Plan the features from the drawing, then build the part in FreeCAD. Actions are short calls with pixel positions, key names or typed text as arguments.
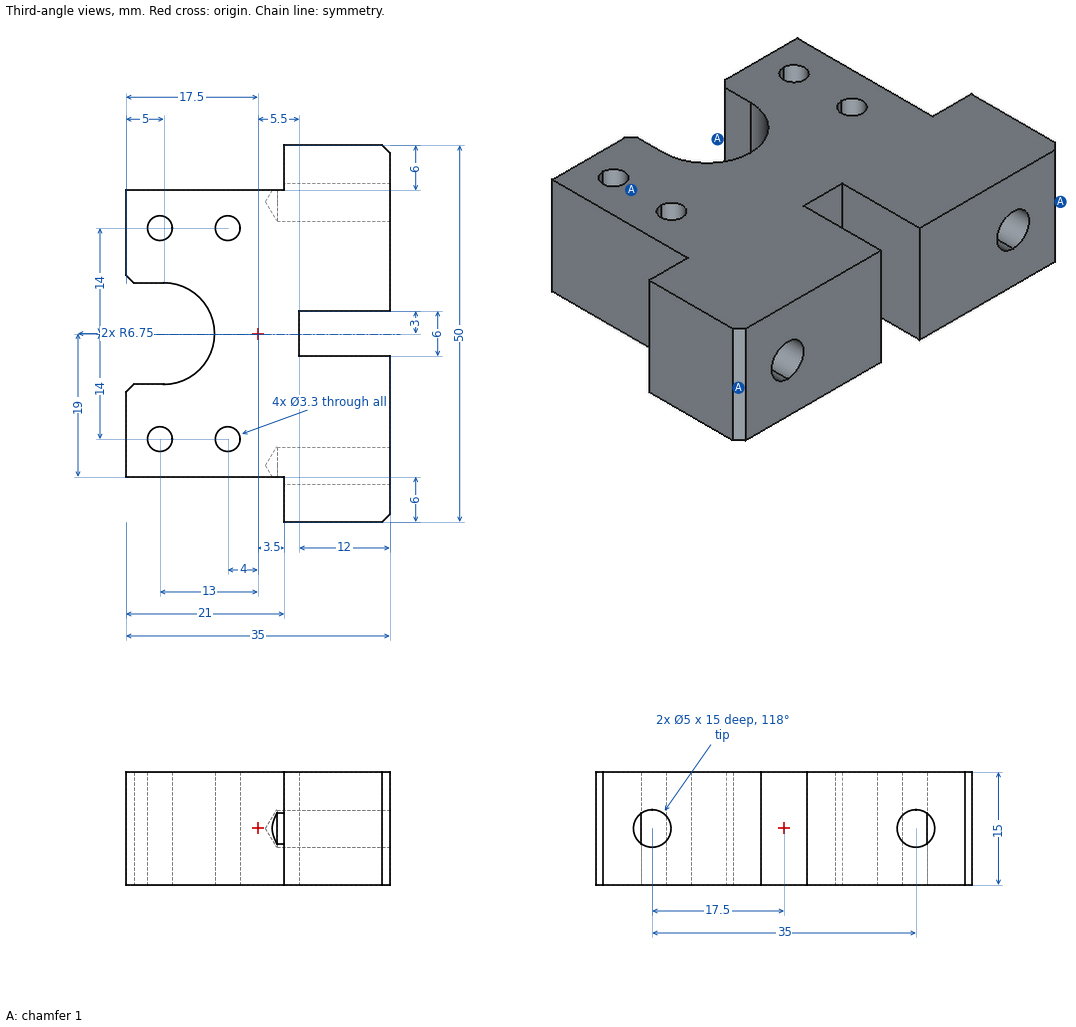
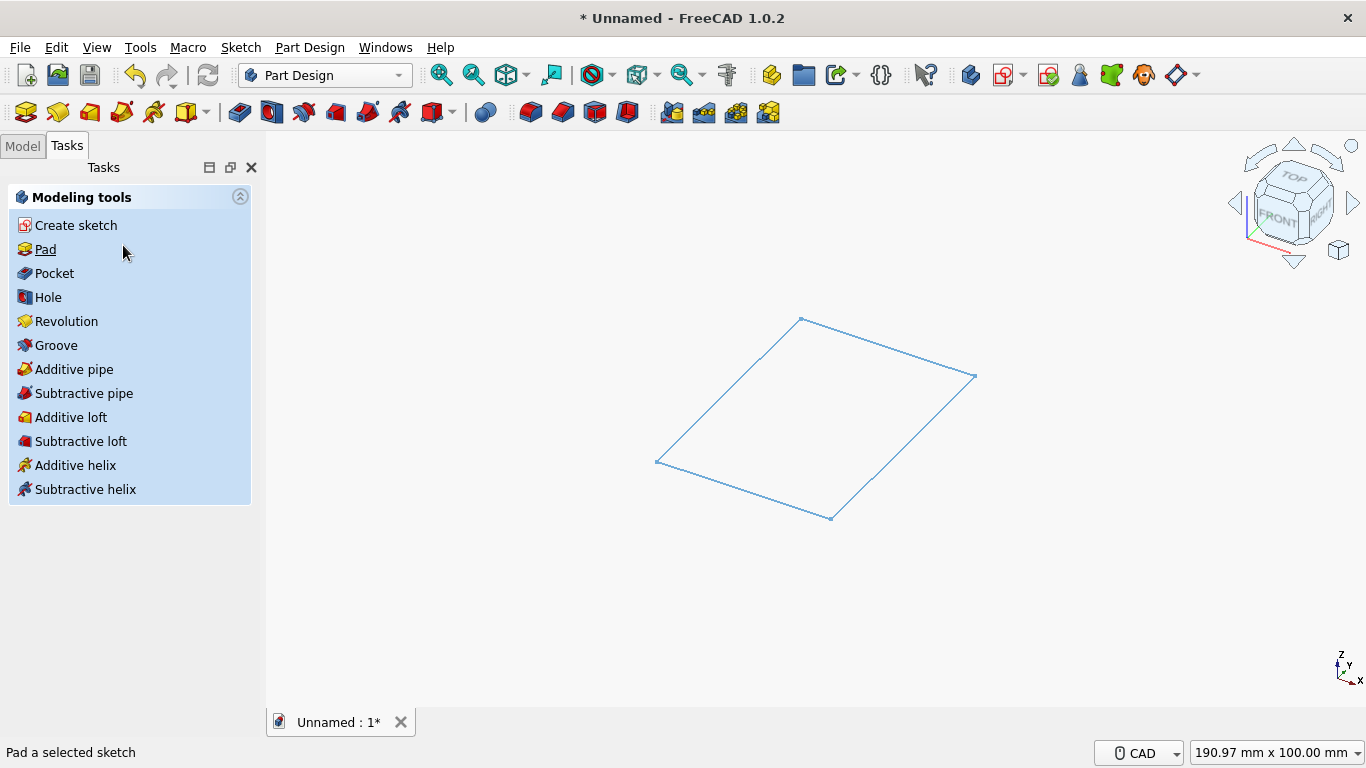
click(26, 112)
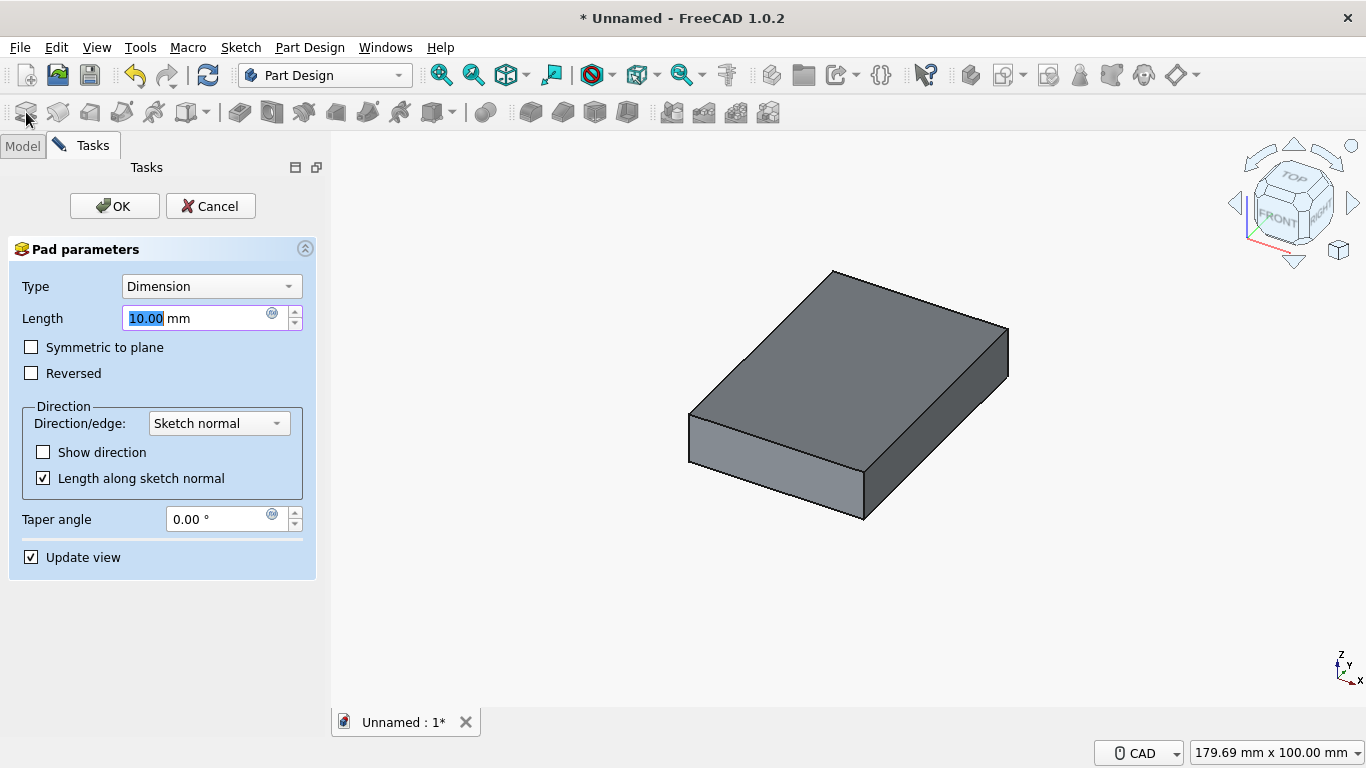
text(15)
key(Tab)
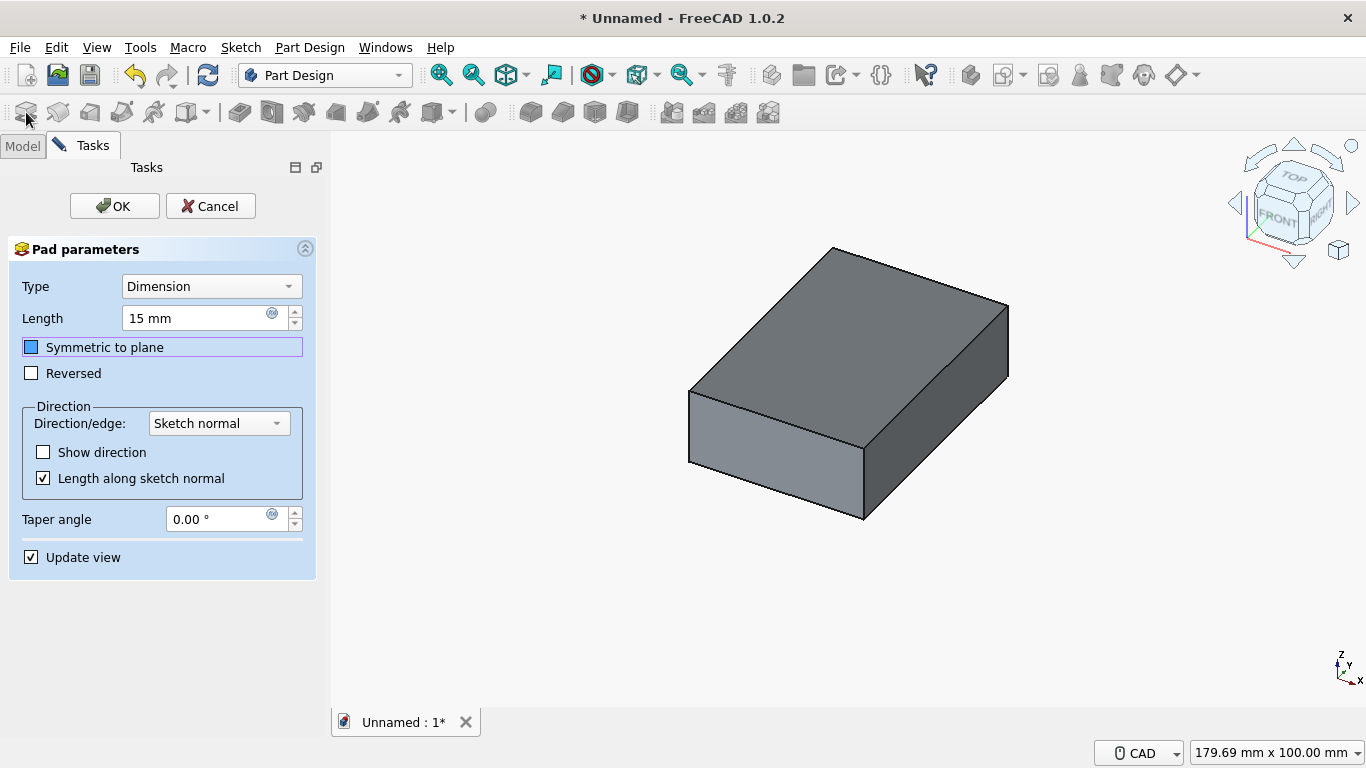
click(30, 347)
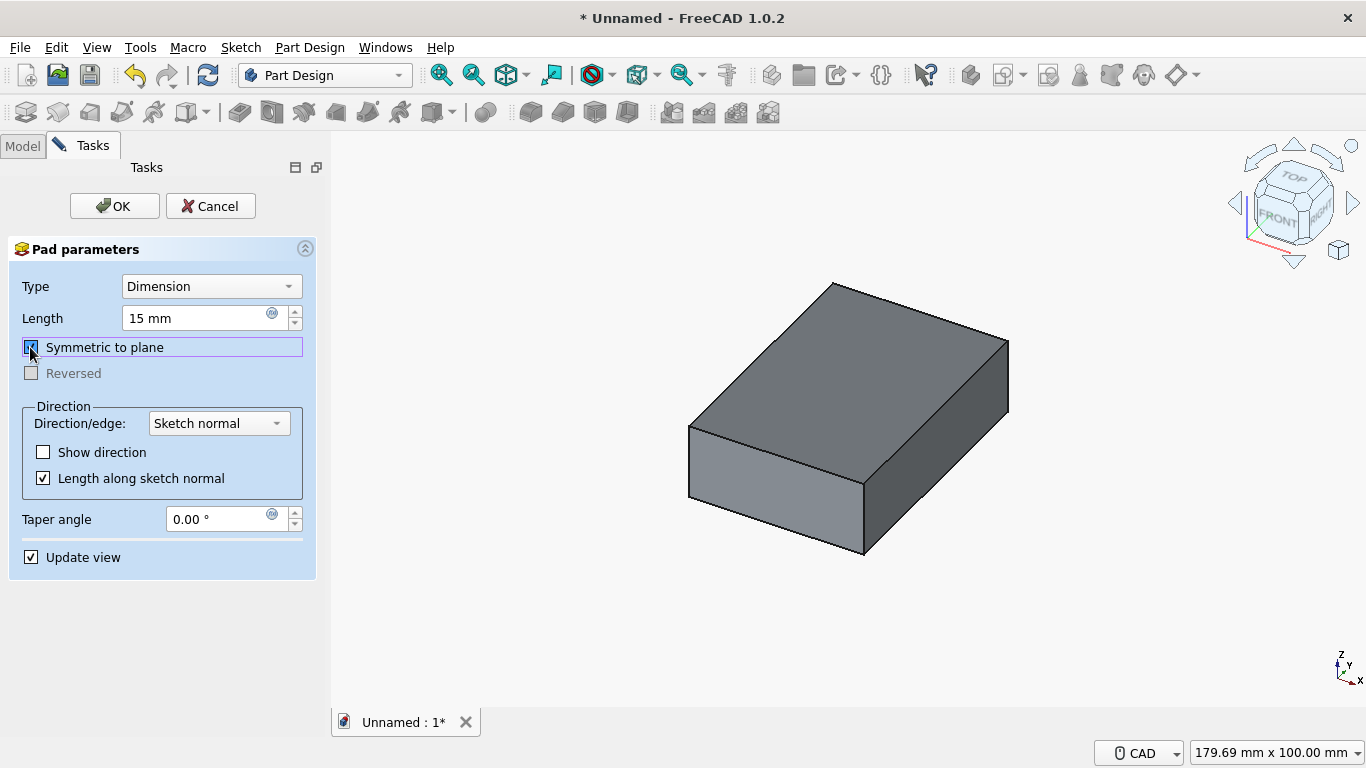
click(115, 206)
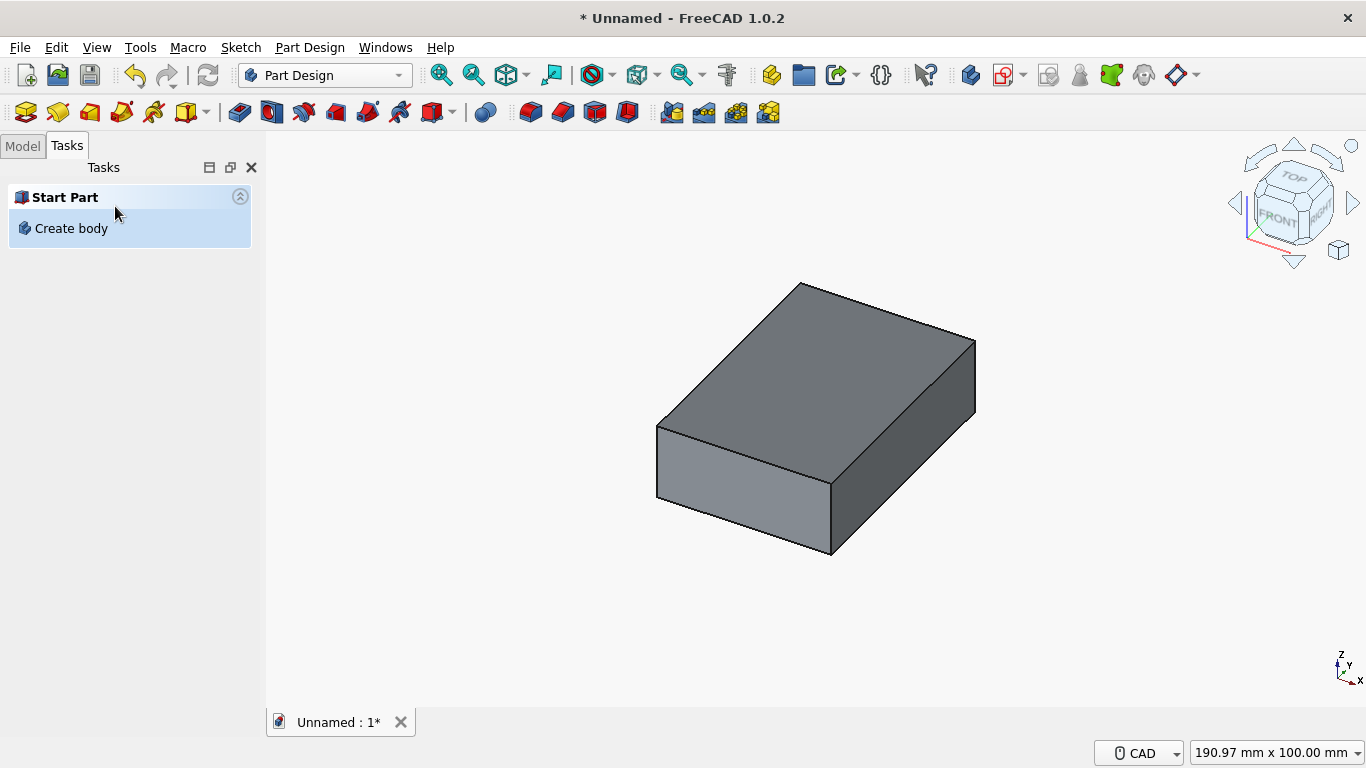
click(837, 362)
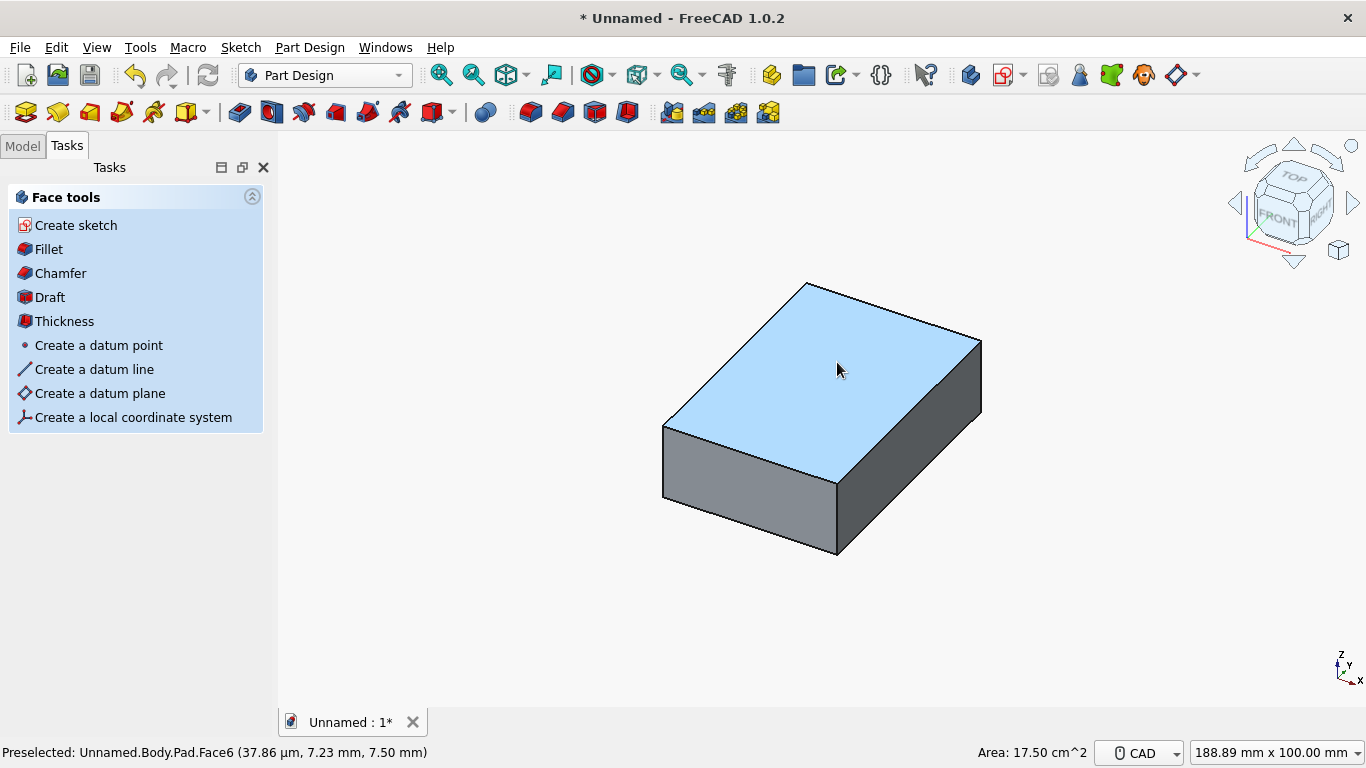
click(1004, 76)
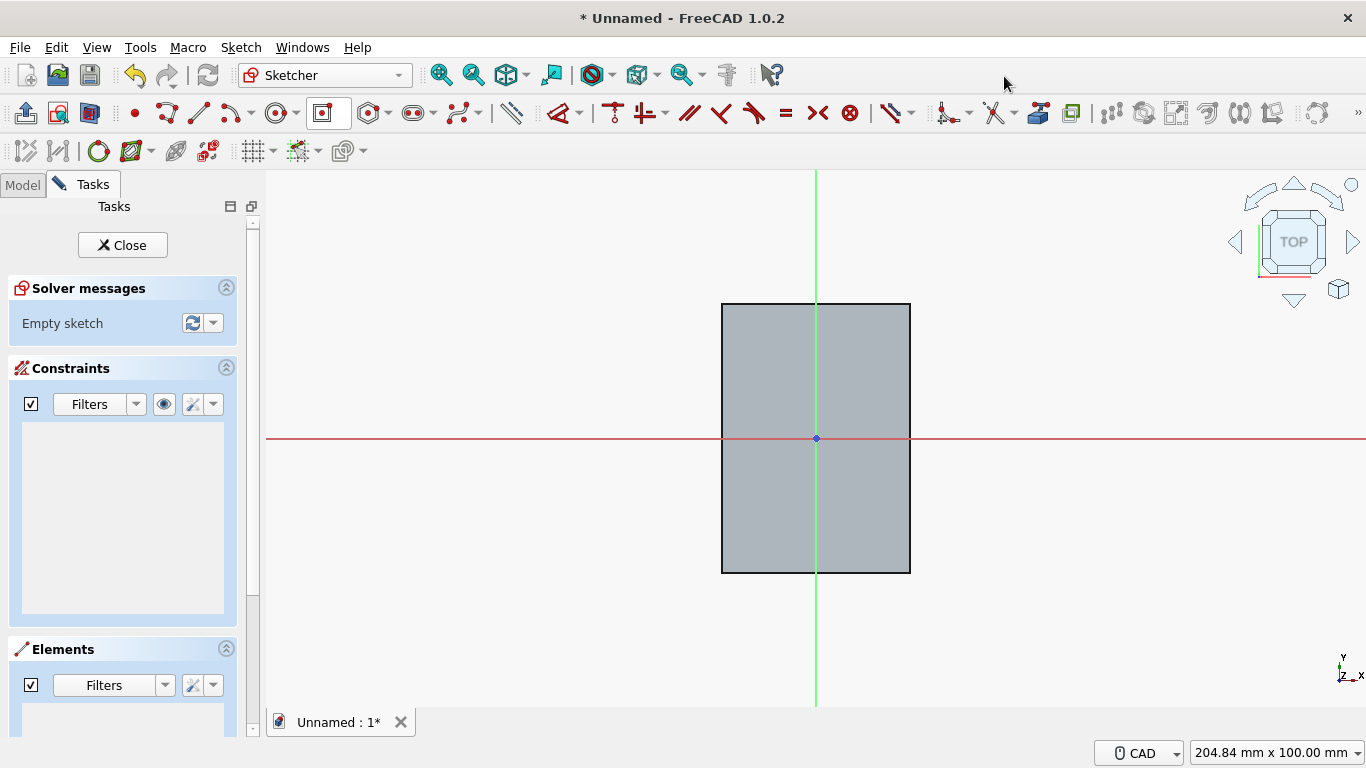
scroll(752, 438, up, 8)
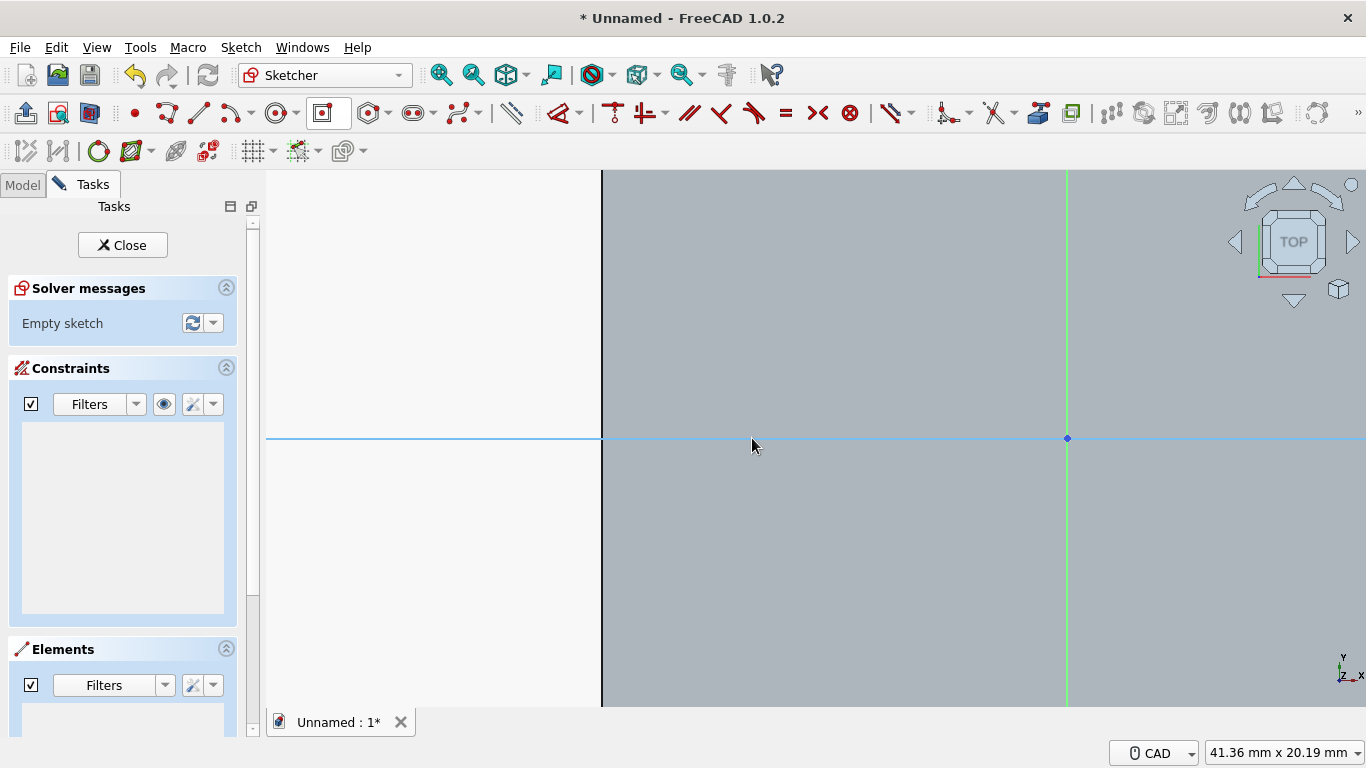
click(414, 114)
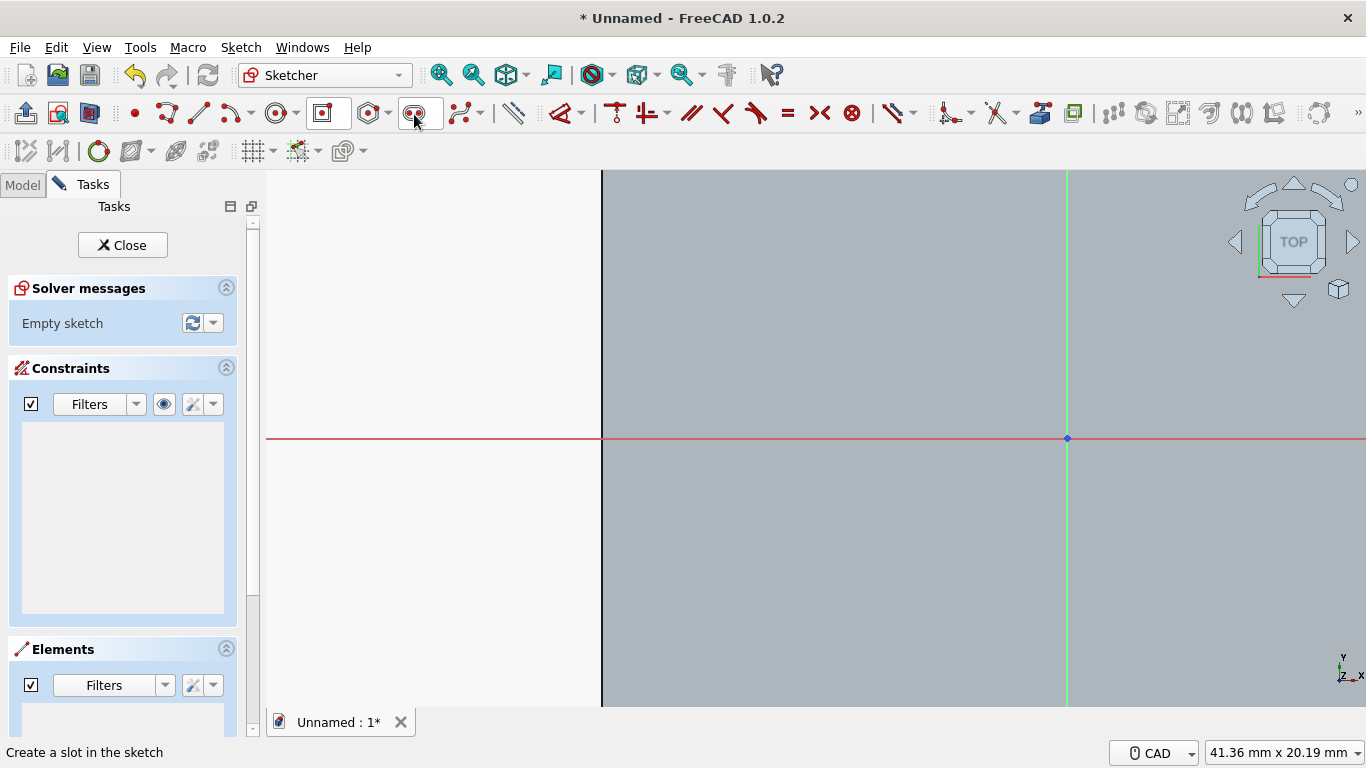
click(602, 438)